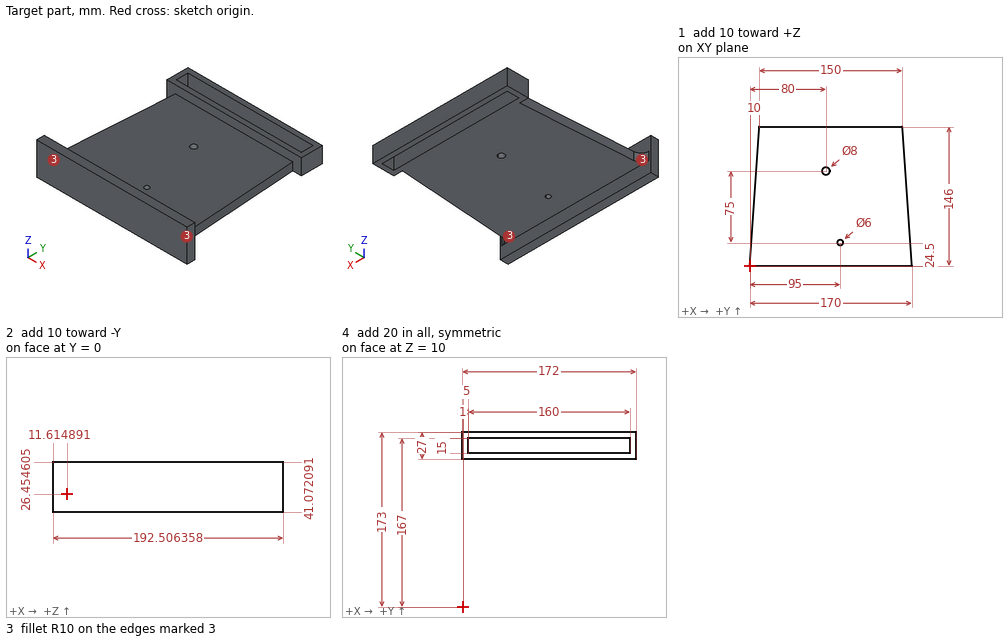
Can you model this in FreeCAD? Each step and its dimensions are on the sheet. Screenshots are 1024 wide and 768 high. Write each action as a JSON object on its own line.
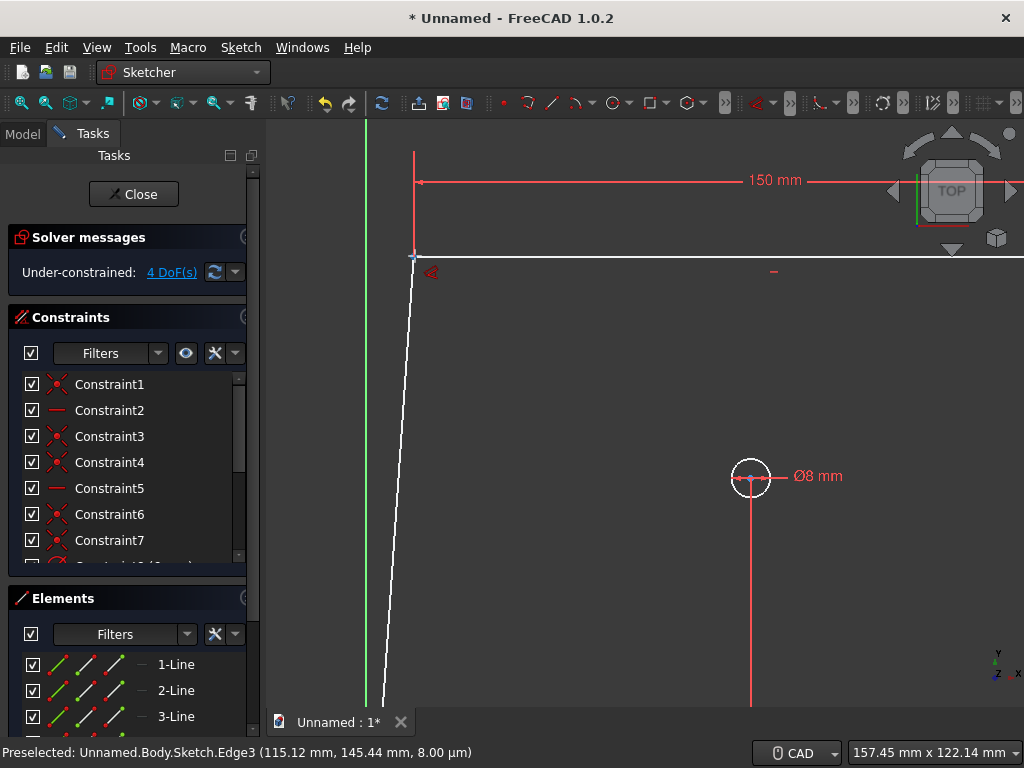
{"action": "left_click", "coordinate": [414, 257]}
{"action": "left_click", "coordinate": [390, 223]}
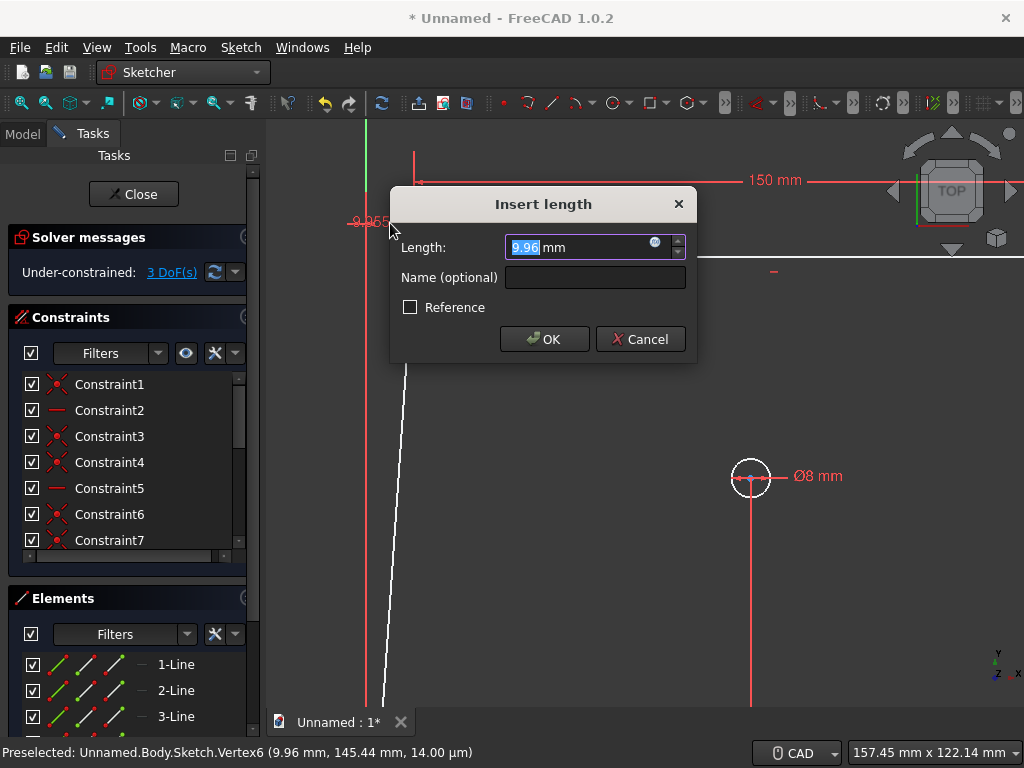
{"action": "type", "text": "10"}
{"action": "key", "text": "Return"}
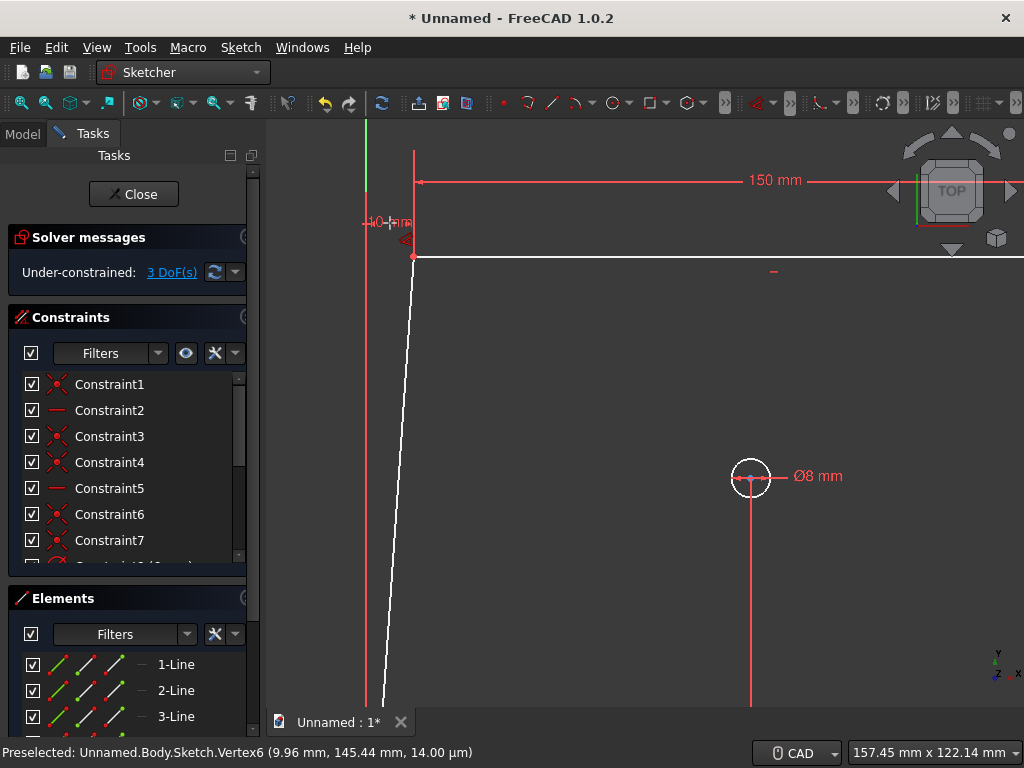
{"action": "scroll", "coordinate": [415, 256], "scroll_direction": "down", "scroll_amount": 4}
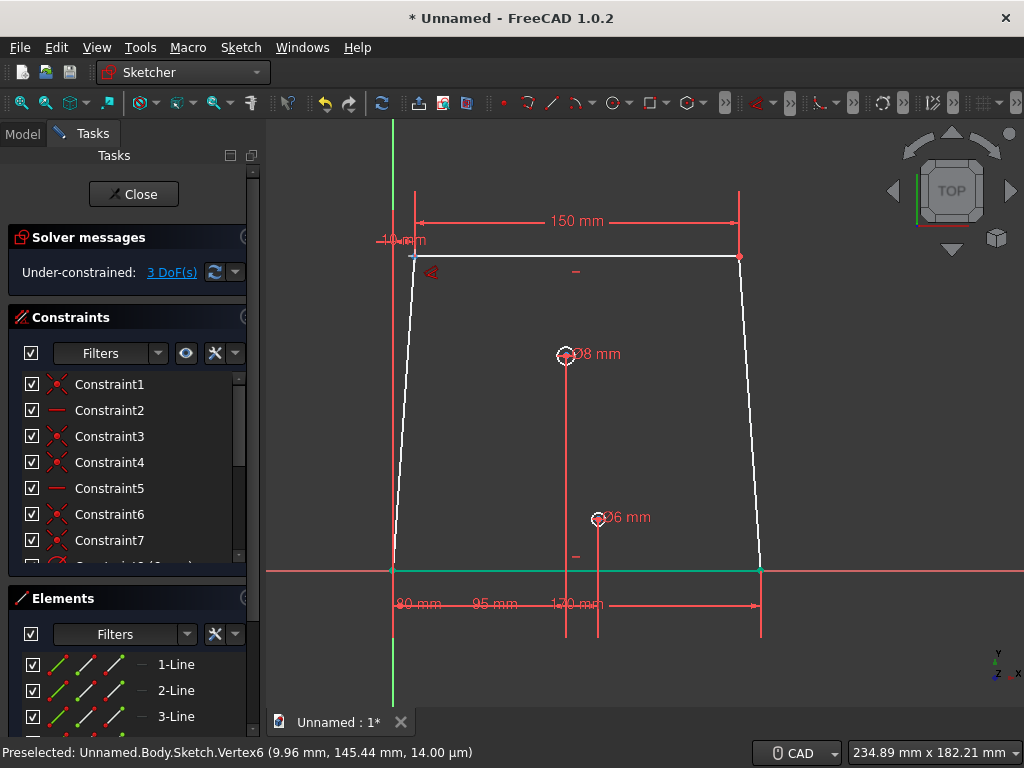
{"action": "left_click", "coordinate": [598, 519]}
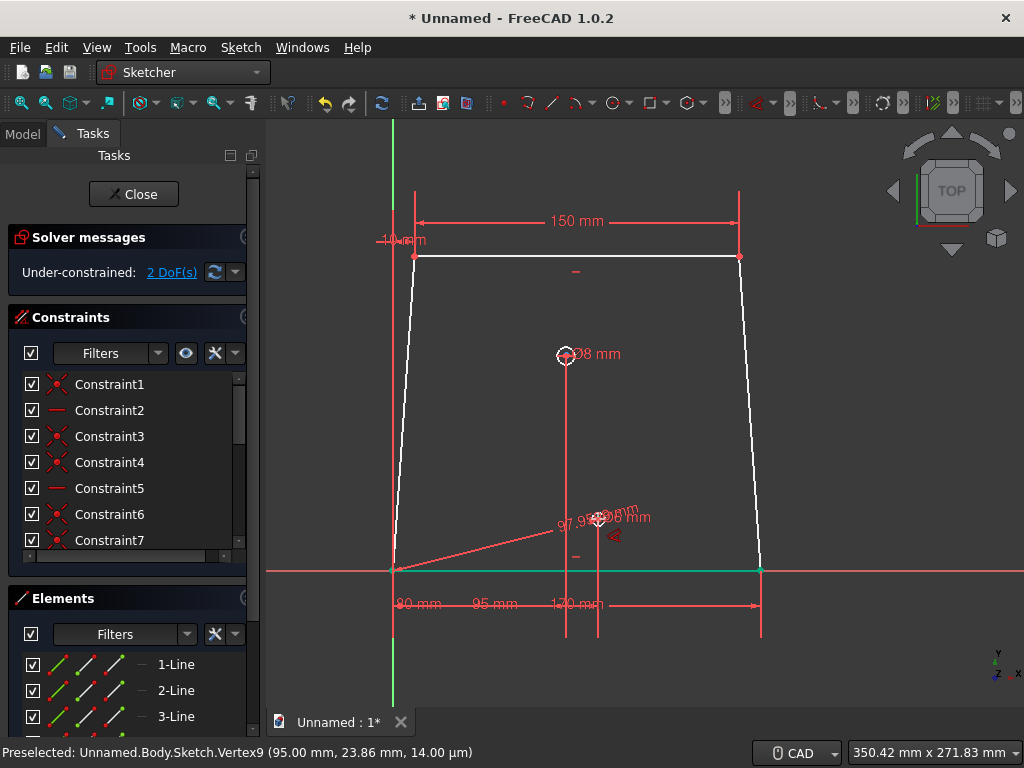
{"action": "left_click", "coordinate": [566, 356]}
{"action": "left_click", "coordinate": [632, 438]}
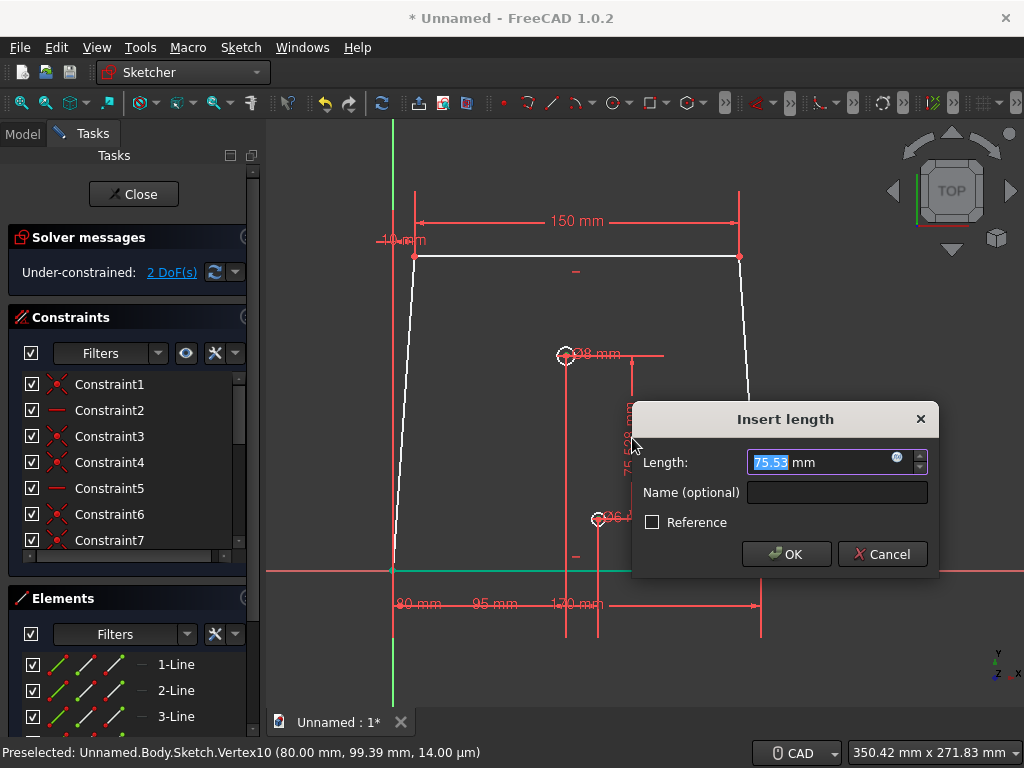
{"action": "type", "text": "75"}
{"action": "key", "text": "Return"}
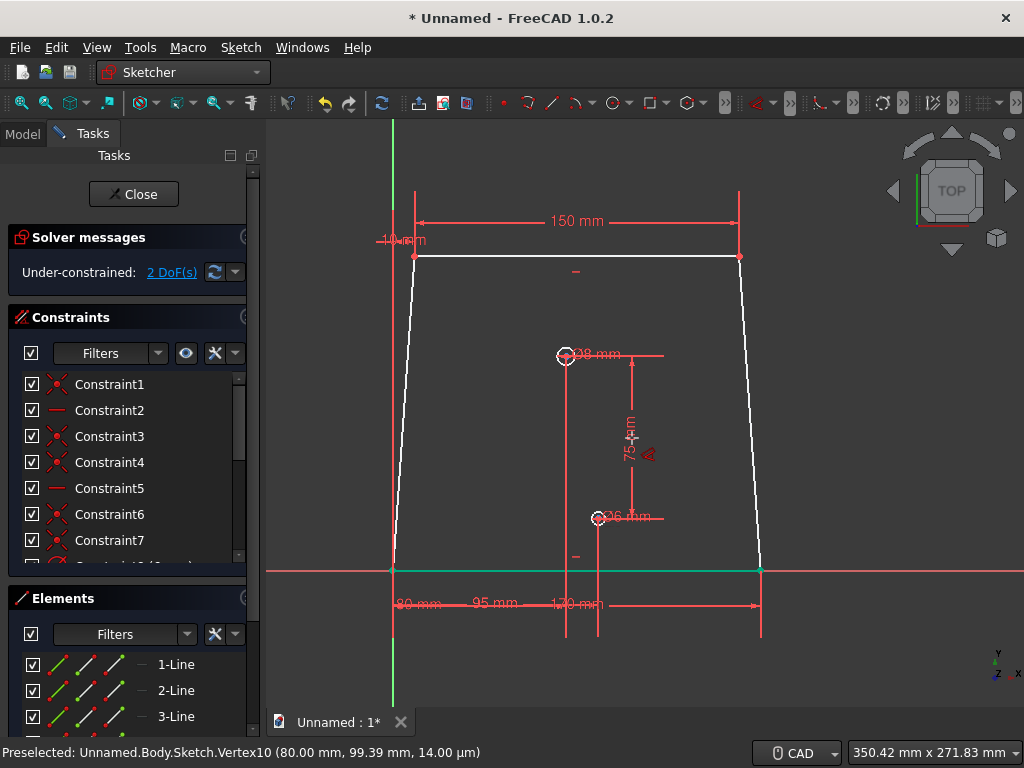
{"action": "left_click", "coordinate": [739, 256]}
{"action": "left_click", "coordinate": [359, 414]}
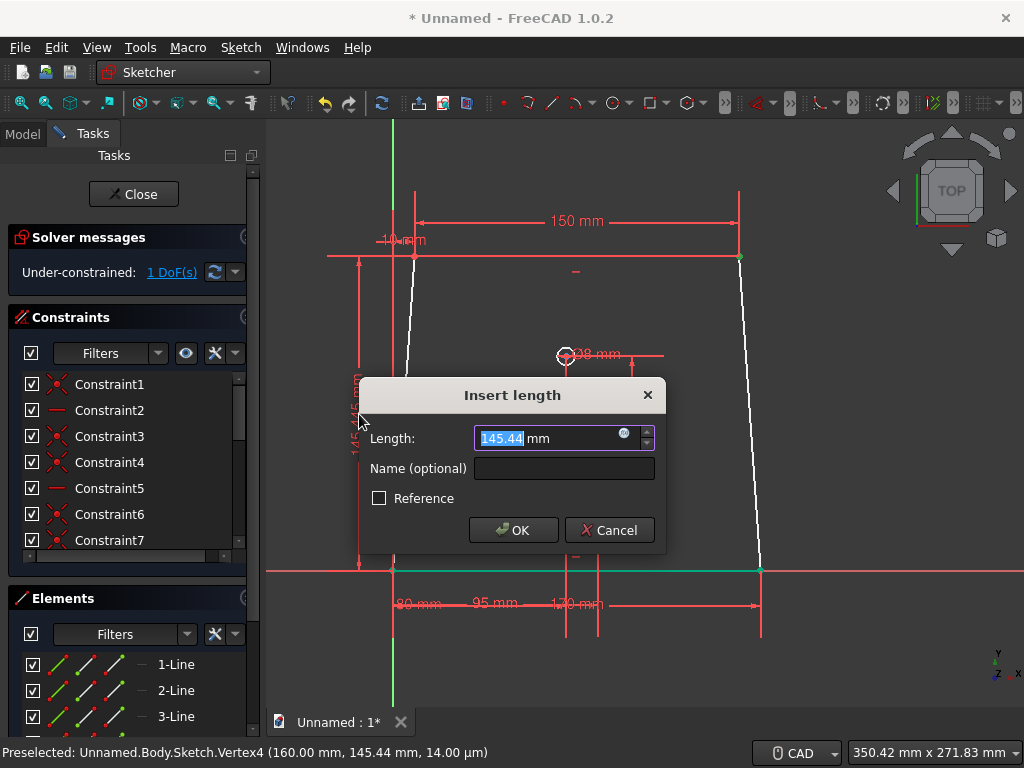
{"action": "type", "text": "146"}
{"action": "key", "text": "Return"}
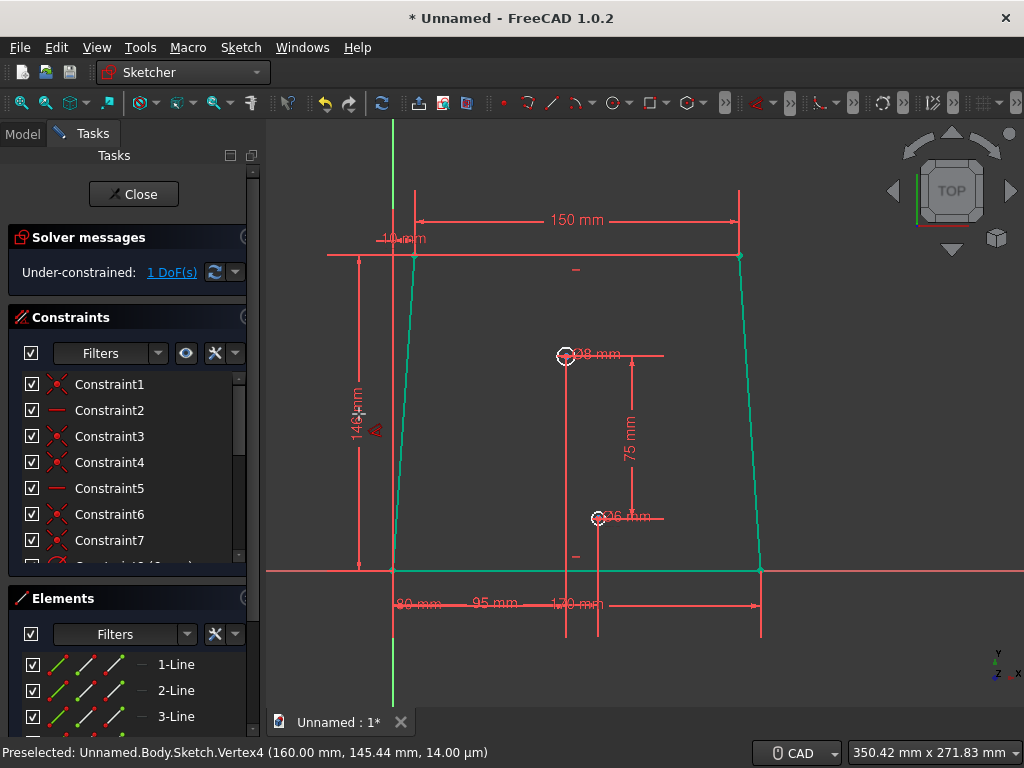
{"action": "left_click", "coordinate": [598, 519]}
{"action": "left_click", "coordinate": [359, 545]}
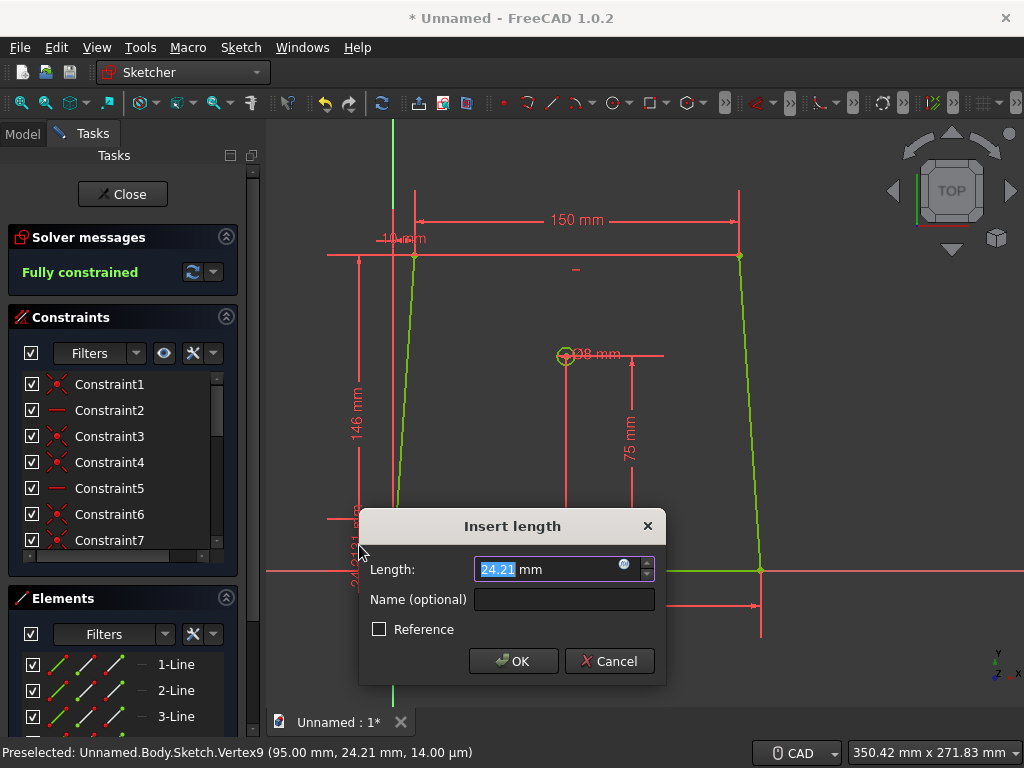
{"action": "type", "text": "24.5"}
{"action": "key", "text": "Return"}
{"action": "key", "text": "Escape"}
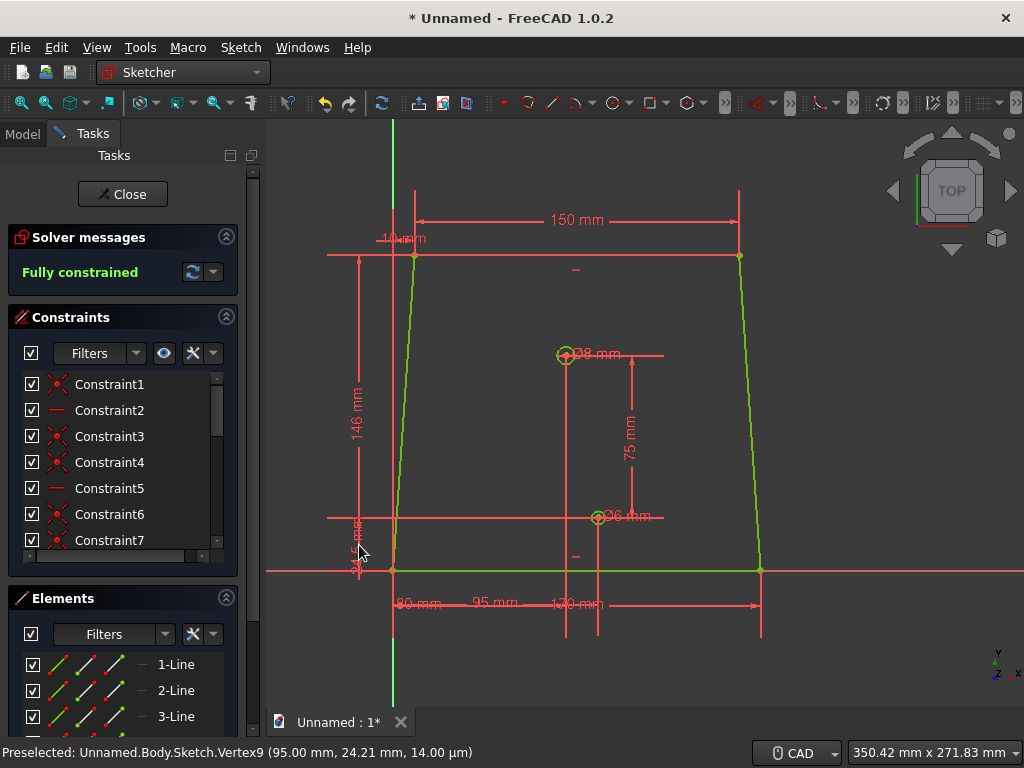
{"action": "left_click", "coordinate": [123, 194]}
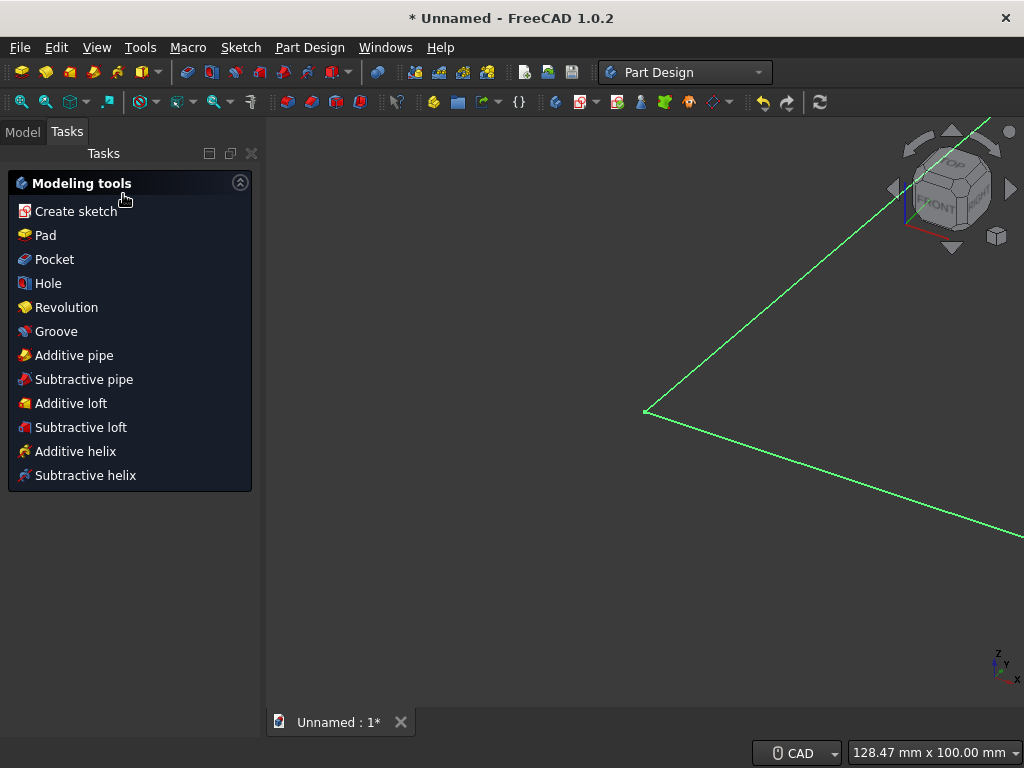
{"action": "left_click", "coordinate": [22, 72]}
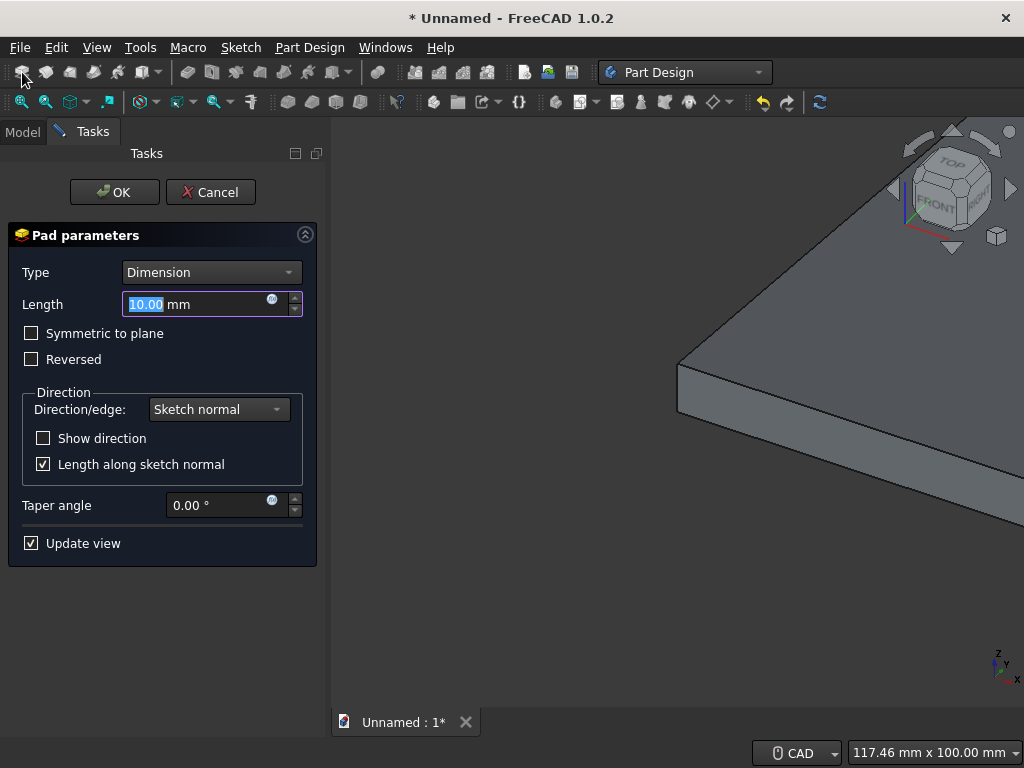
{"action": "type", "text": "10"}
{"action": "key", "text": "Tab"}